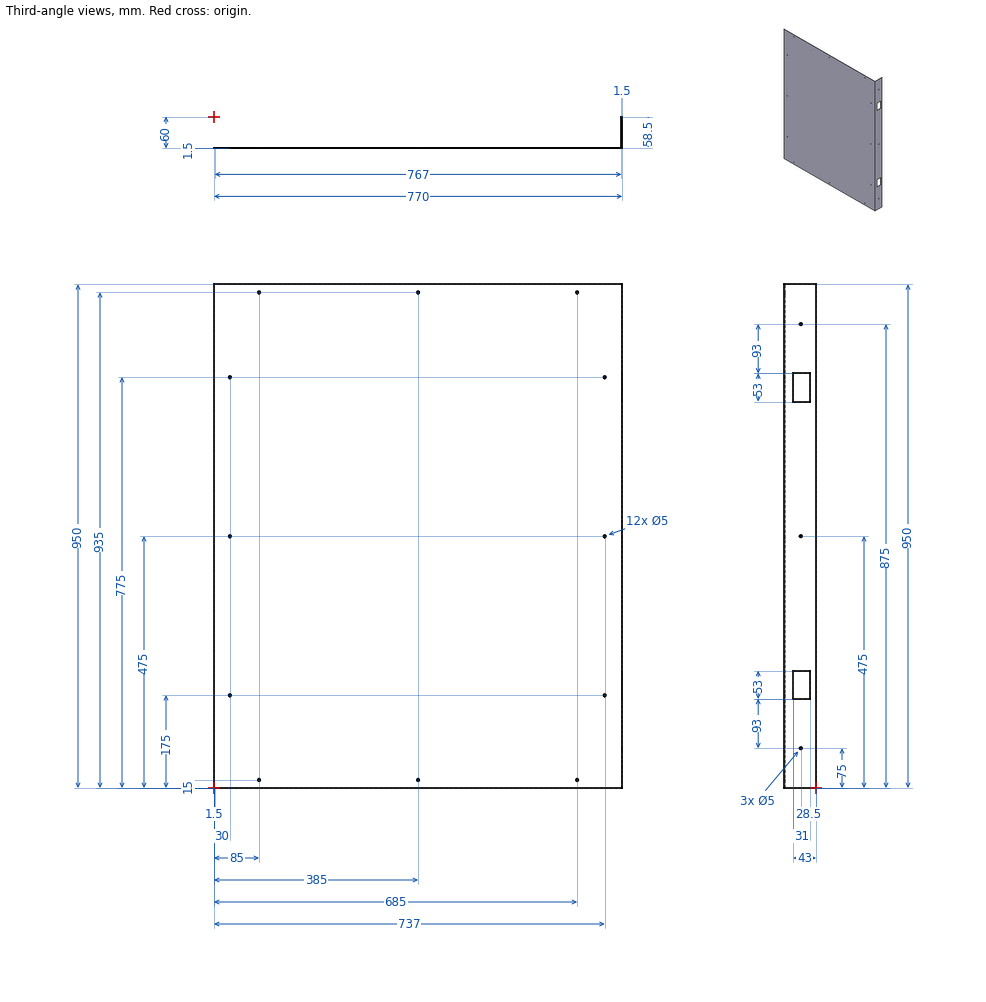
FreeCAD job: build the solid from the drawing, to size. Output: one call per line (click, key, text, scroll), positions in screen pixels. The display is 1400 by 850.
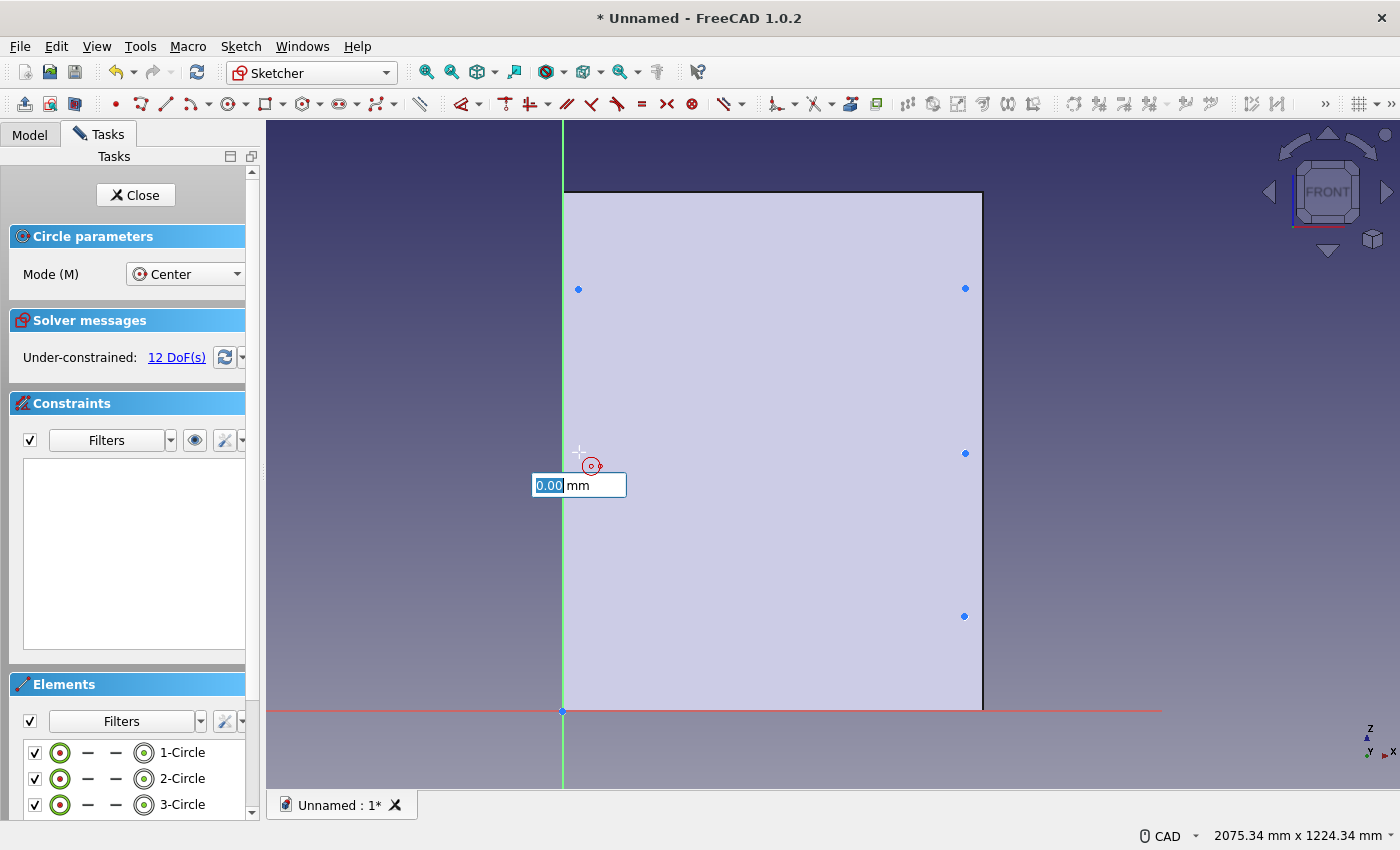
scroll(580, 451, up, 13)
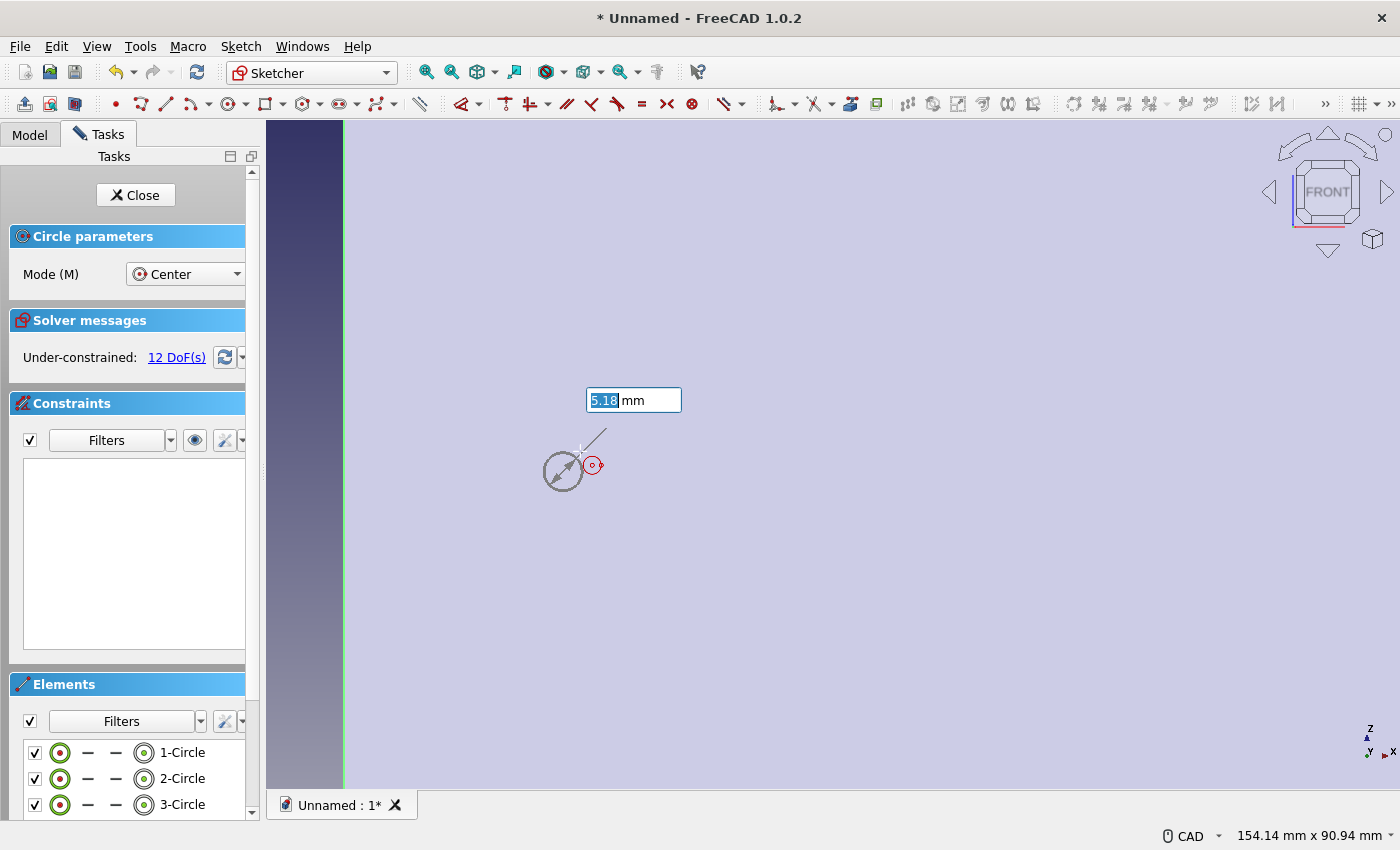
click(578, 442)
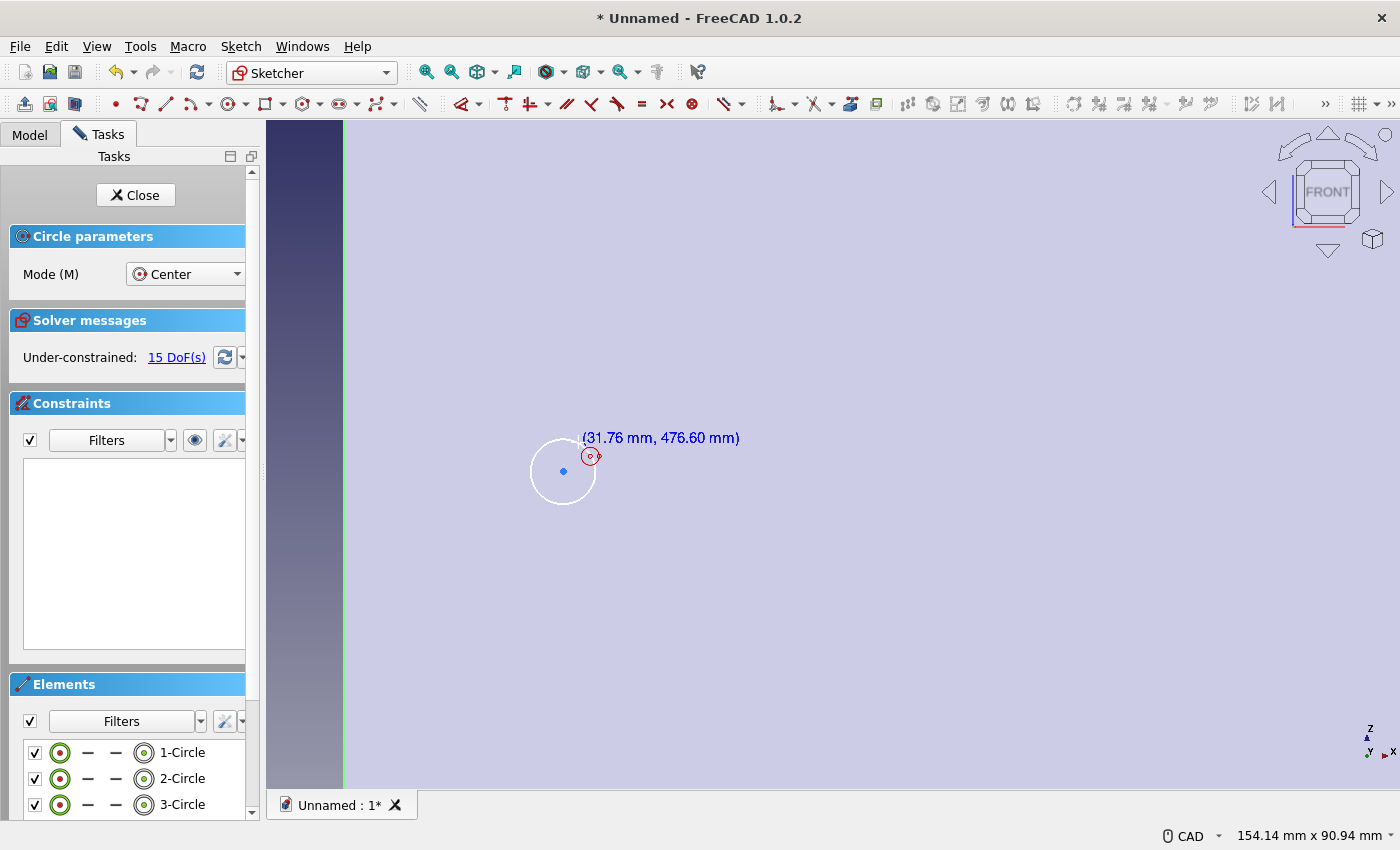
scroll(616, 452, down, 14)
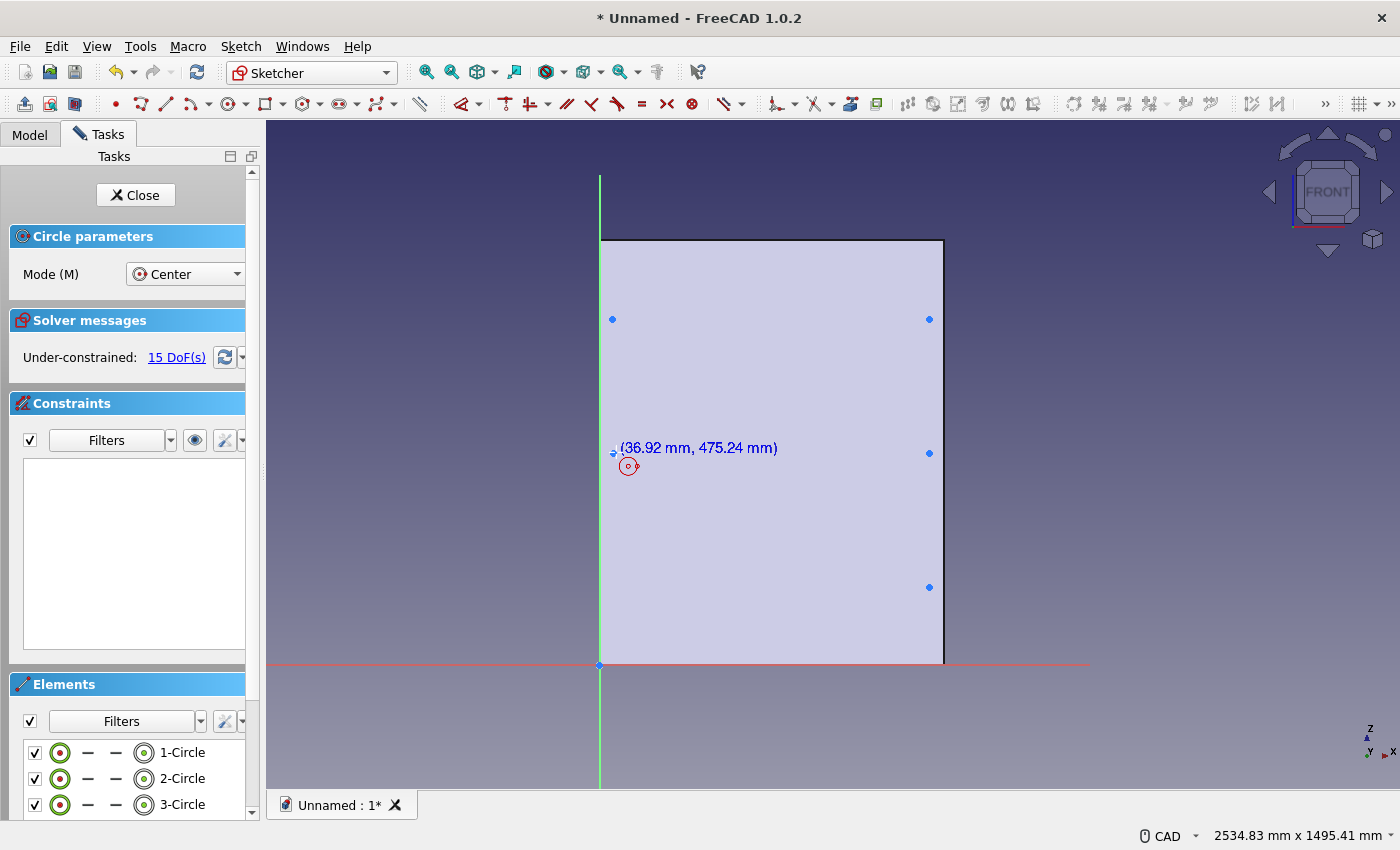
scroll(613, 587, up, 16)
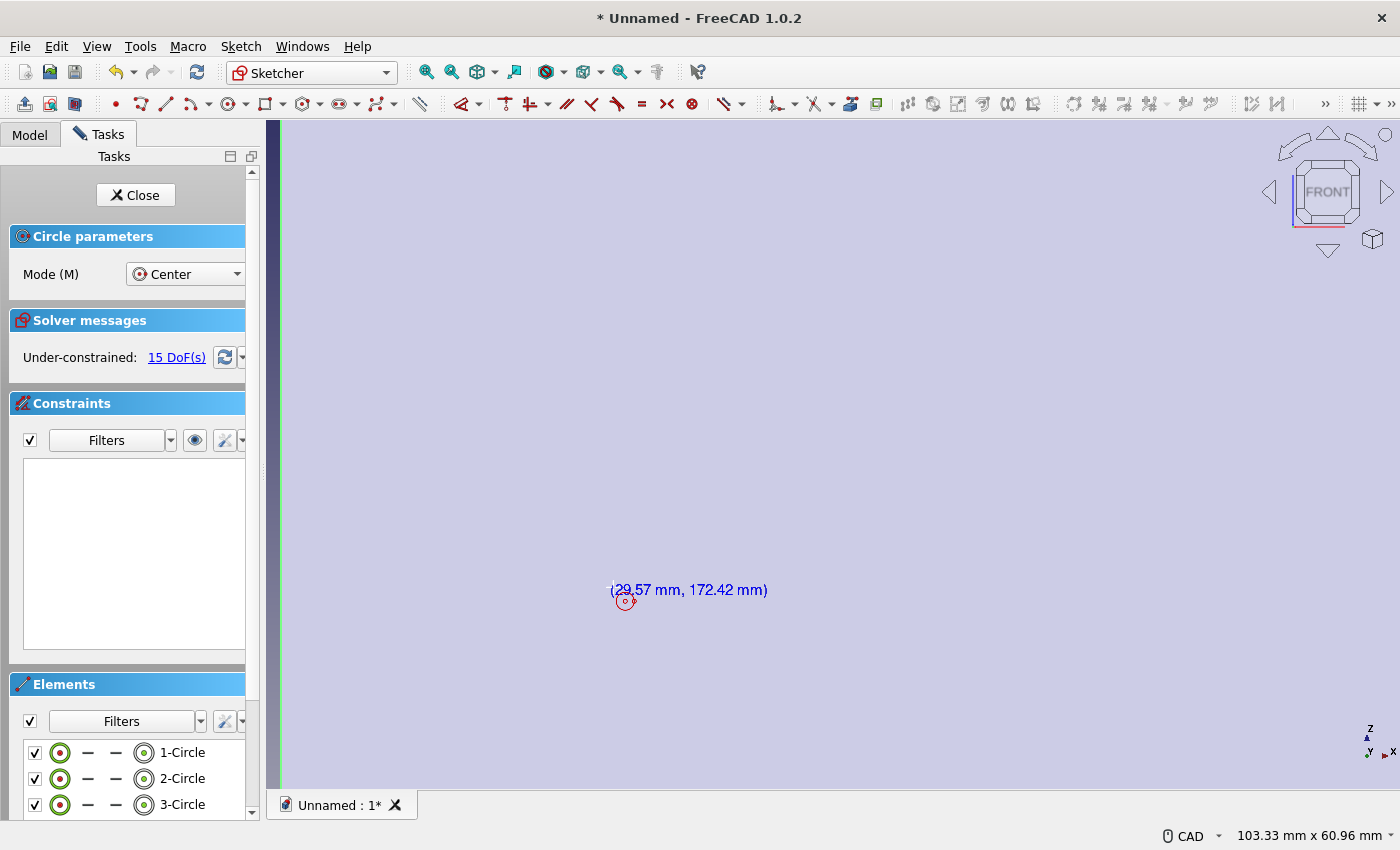
scroll(577, 618, down, 15)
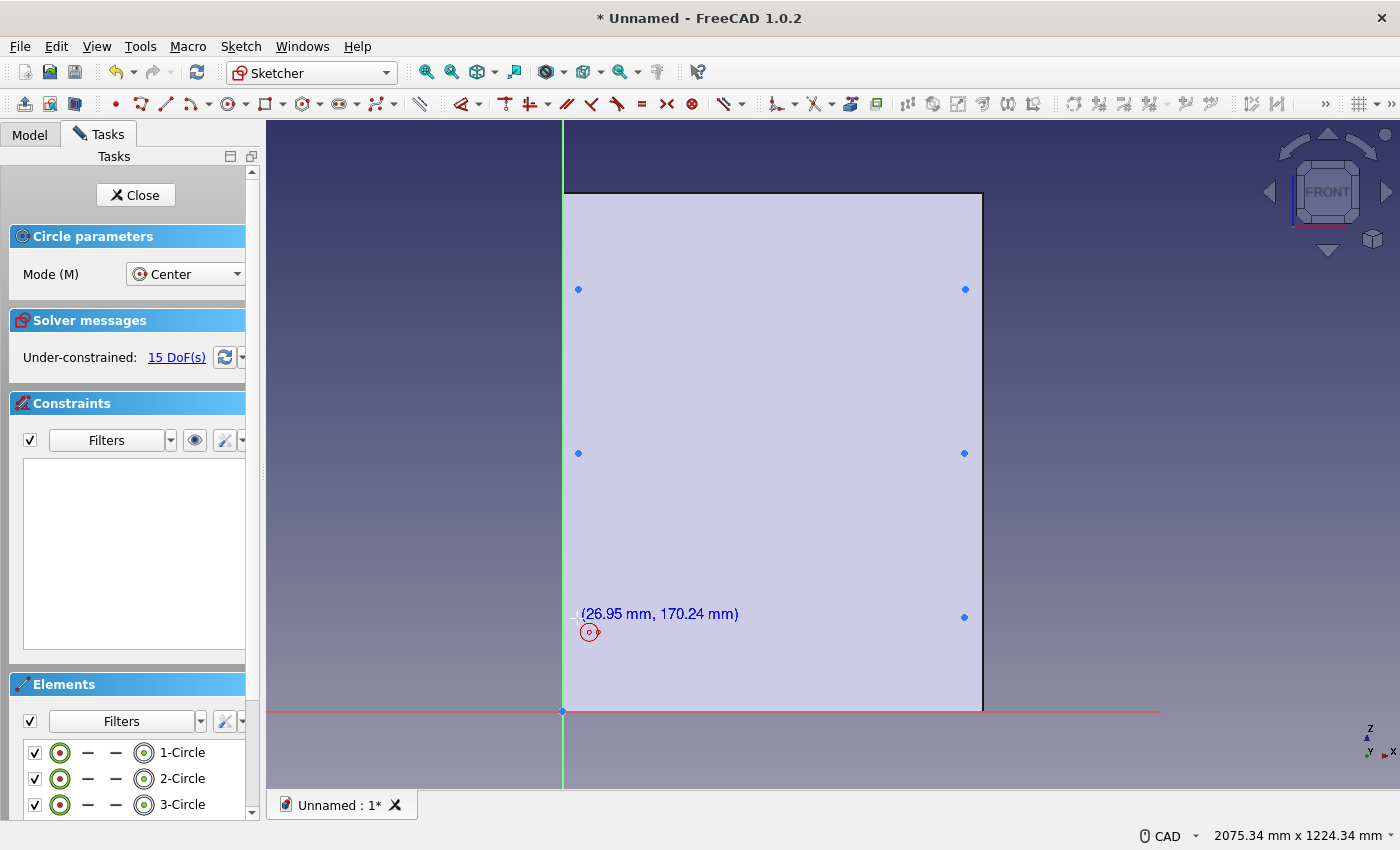
click(579, 616)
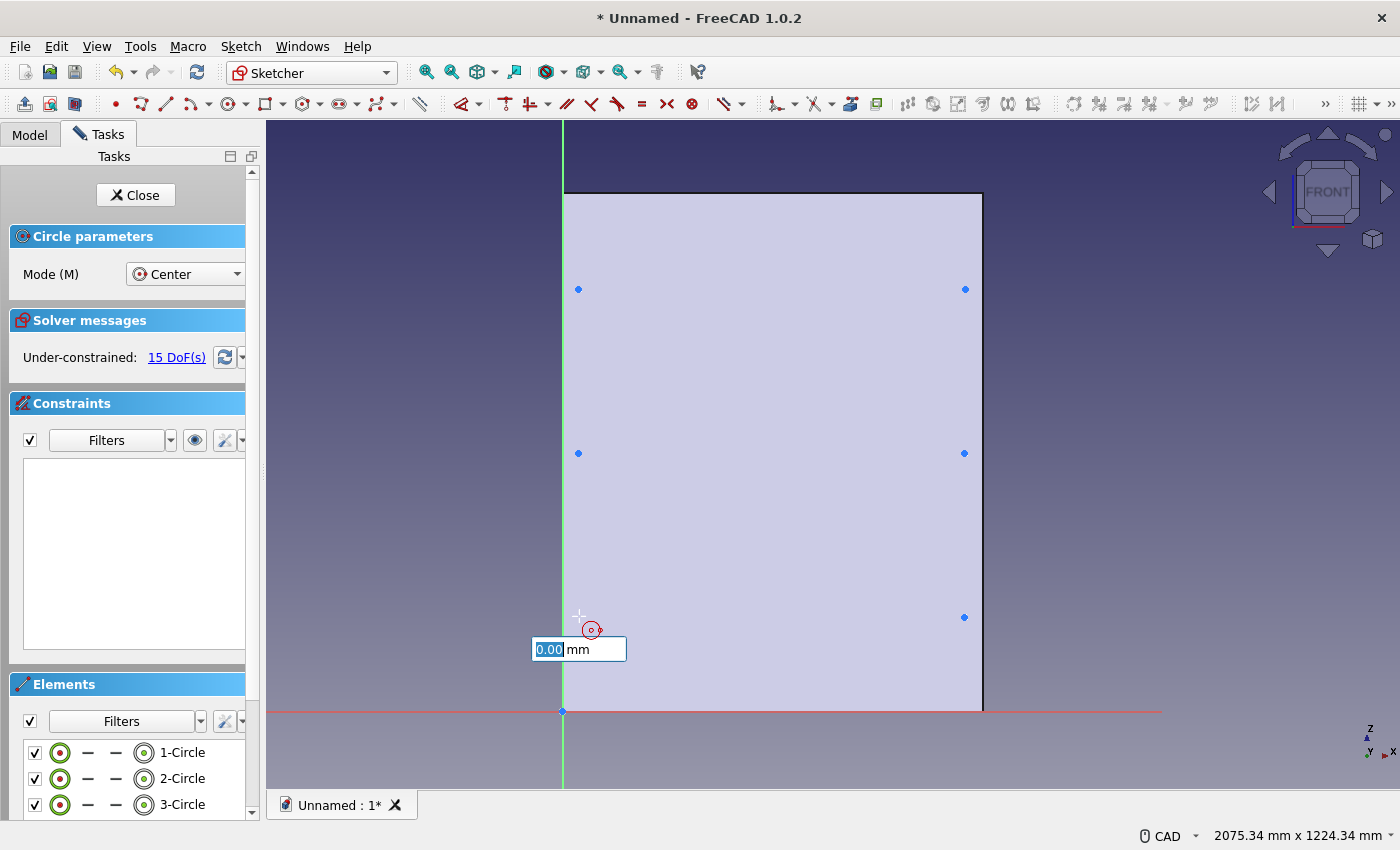
scroll(580, 615, up, 13)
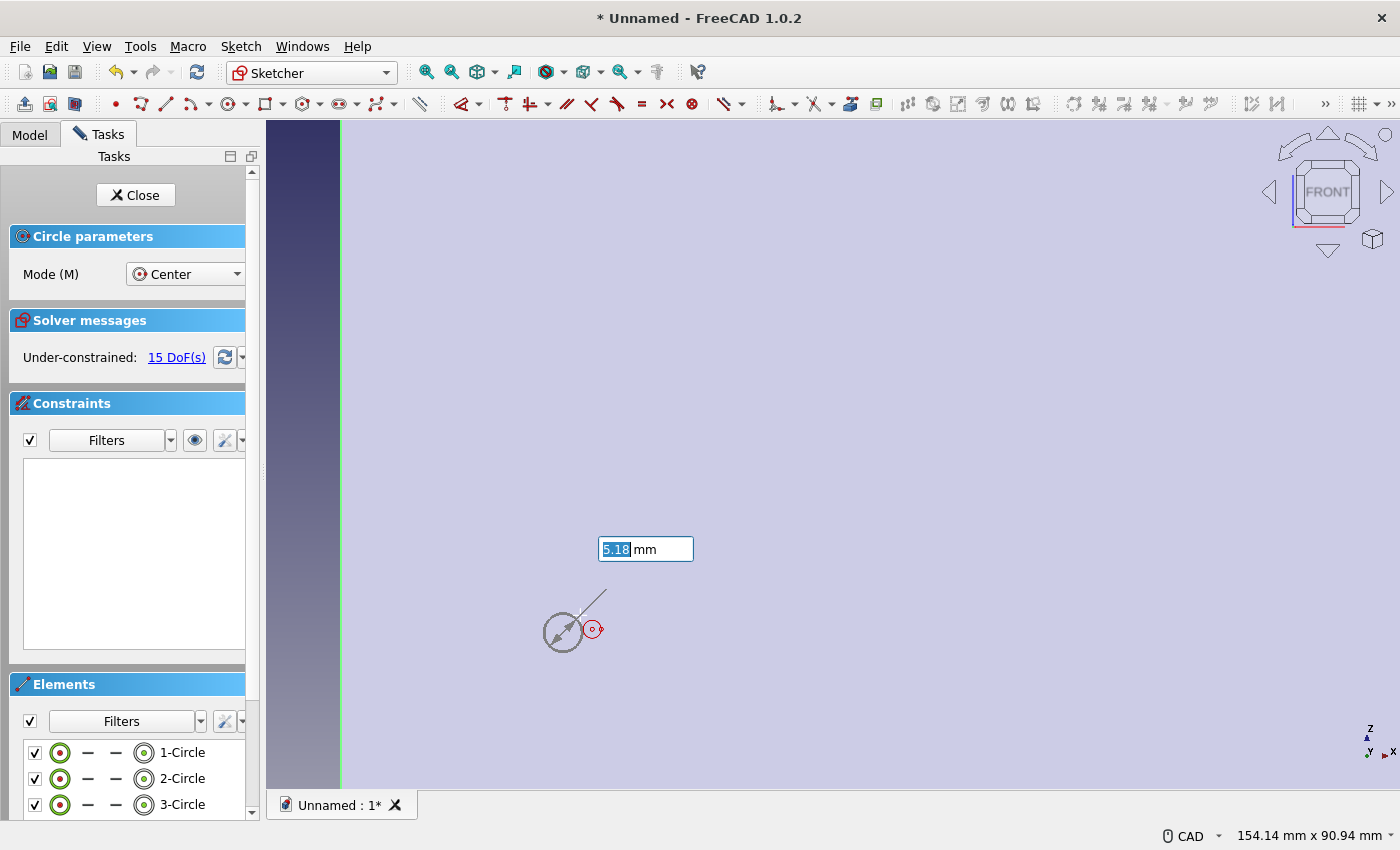
click(575, 608)